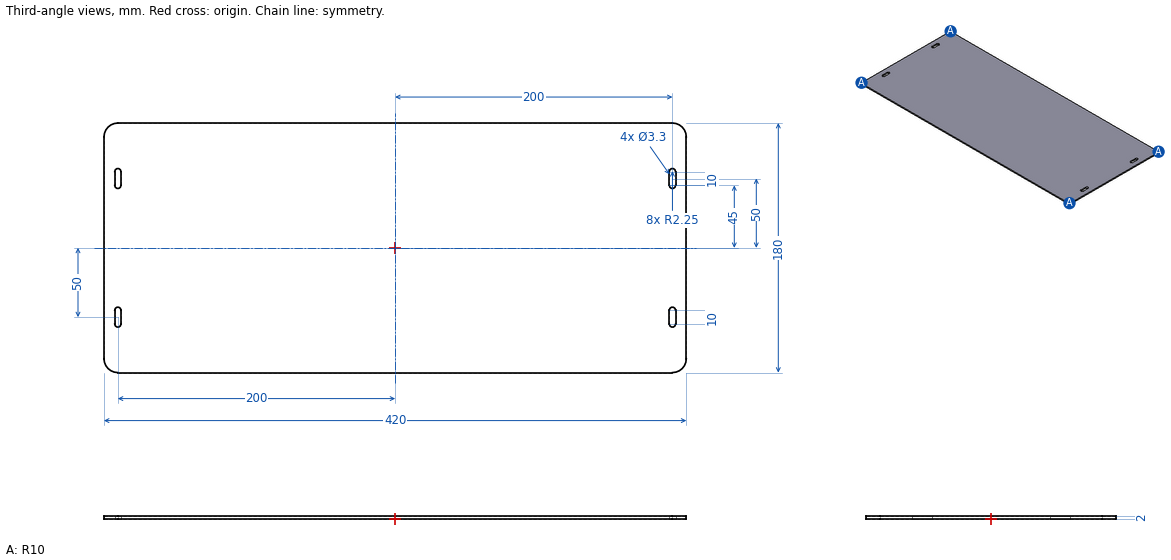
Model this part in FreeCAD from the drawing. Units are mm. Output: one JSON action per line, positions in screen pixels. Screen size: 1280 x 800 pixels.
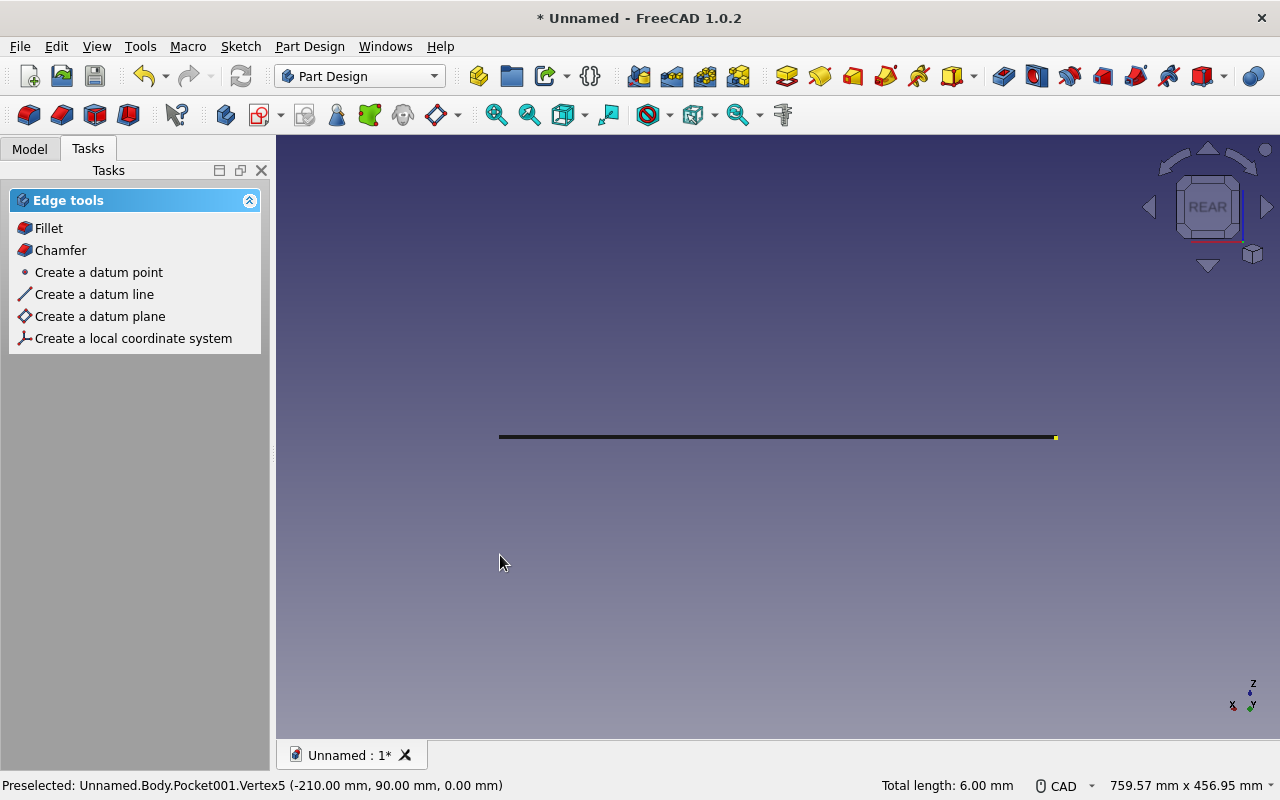
{"action": "scroll", "coordinate": [1056, 436], "scroll_direction": "up", "scroll_amount": 14}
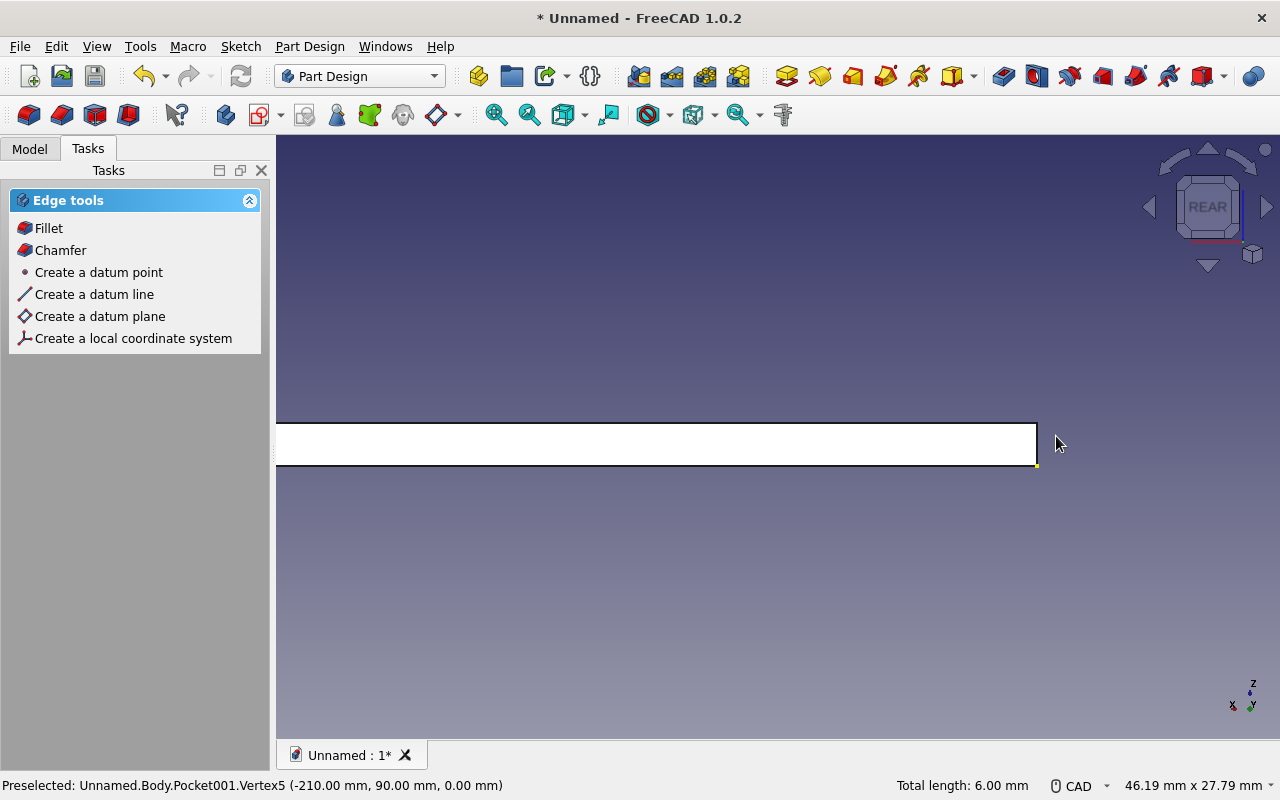
{"action": "left_click", "coordinate": [1037, 444], "text": "ctrl"}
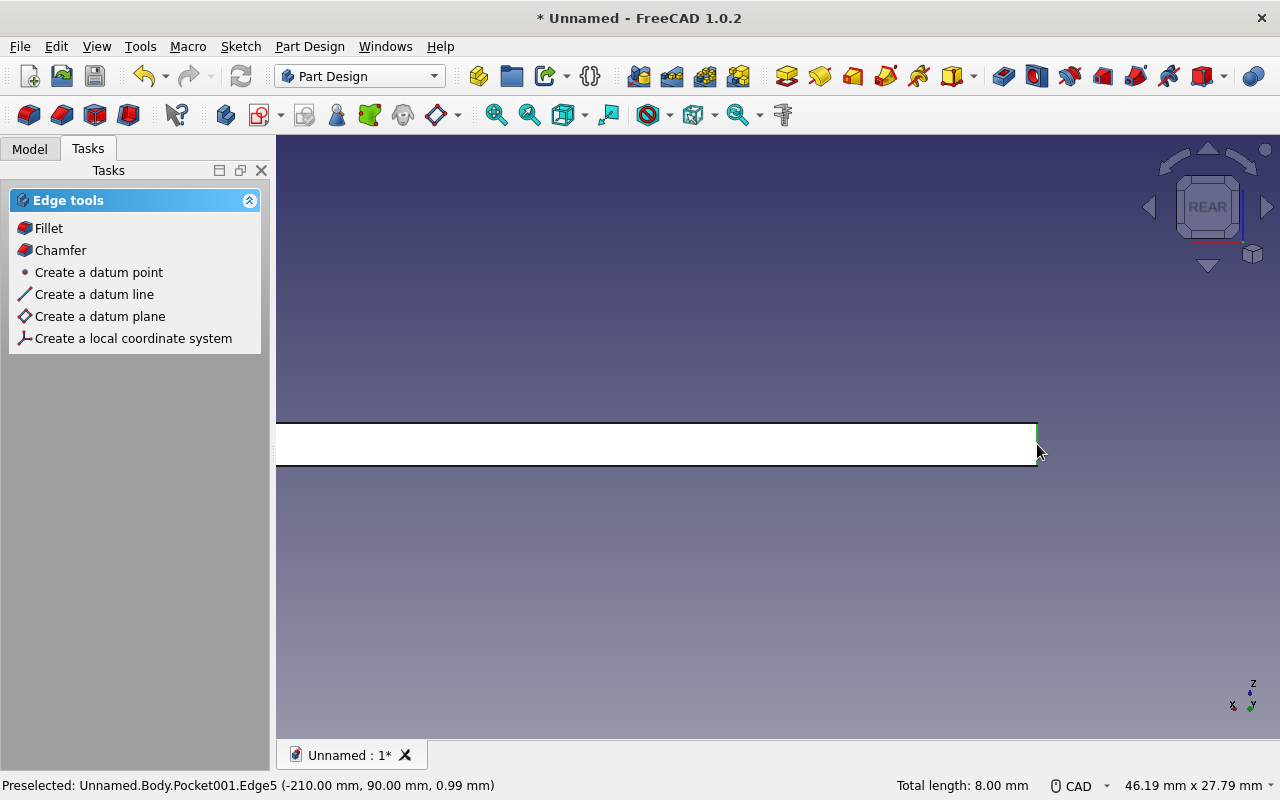
{"action": "left_click", "coordinate": [29, 116]}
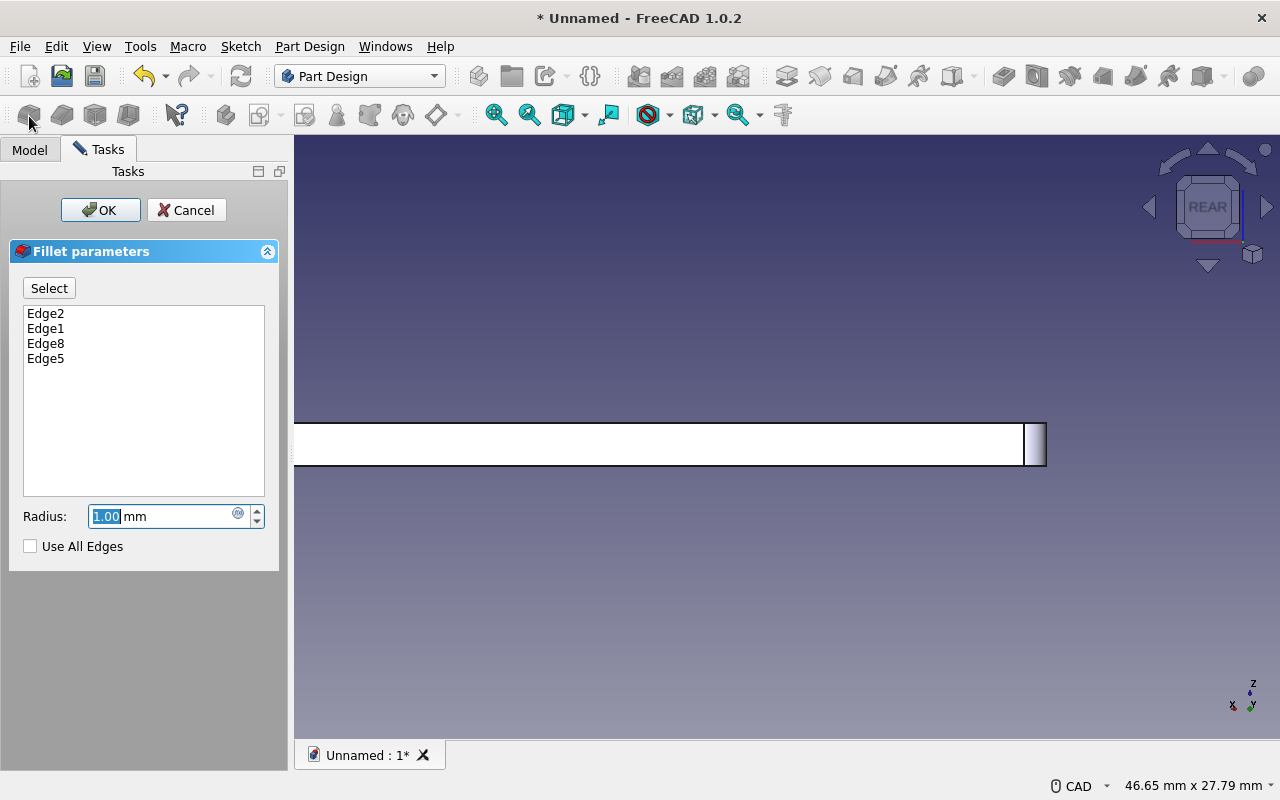
{"action": "type", "text": "10"}
{"action": "key", "text": "Tab"}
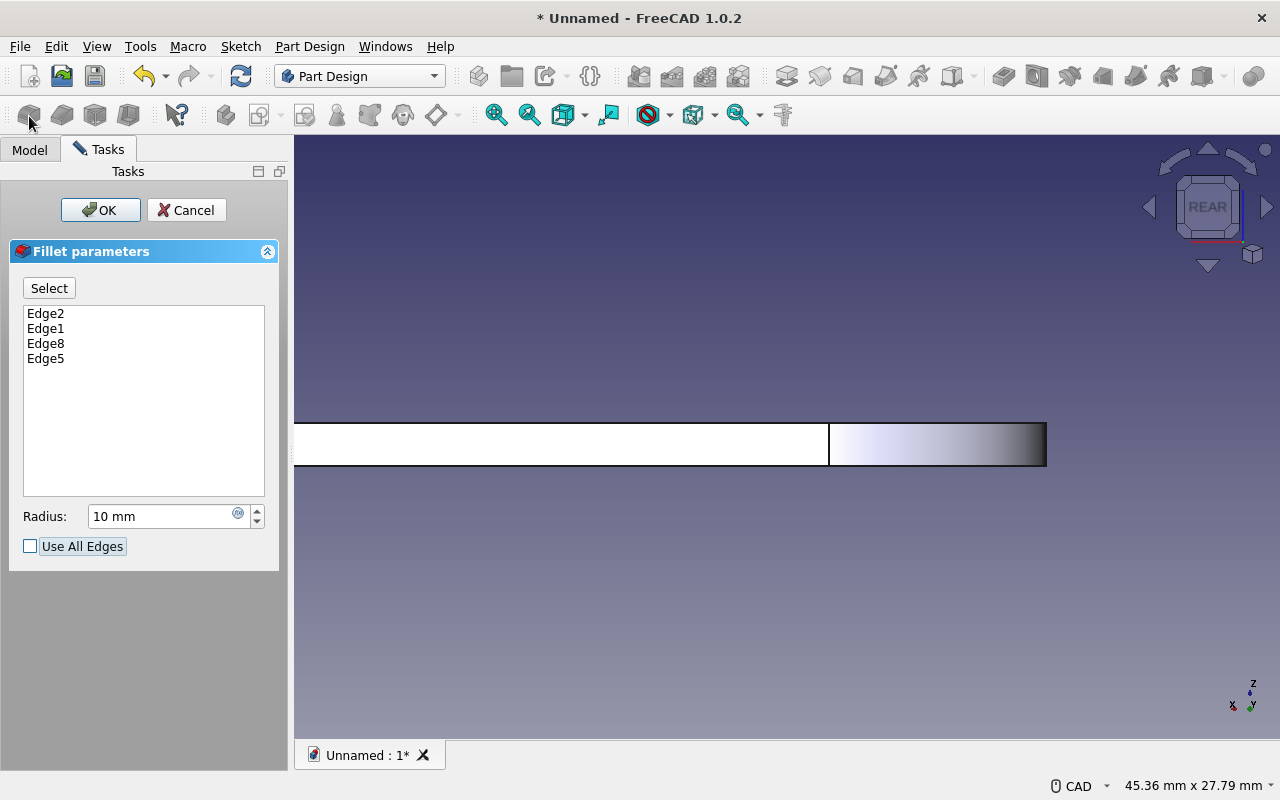
{"action": "left_click", "coordinate": [101, 210]}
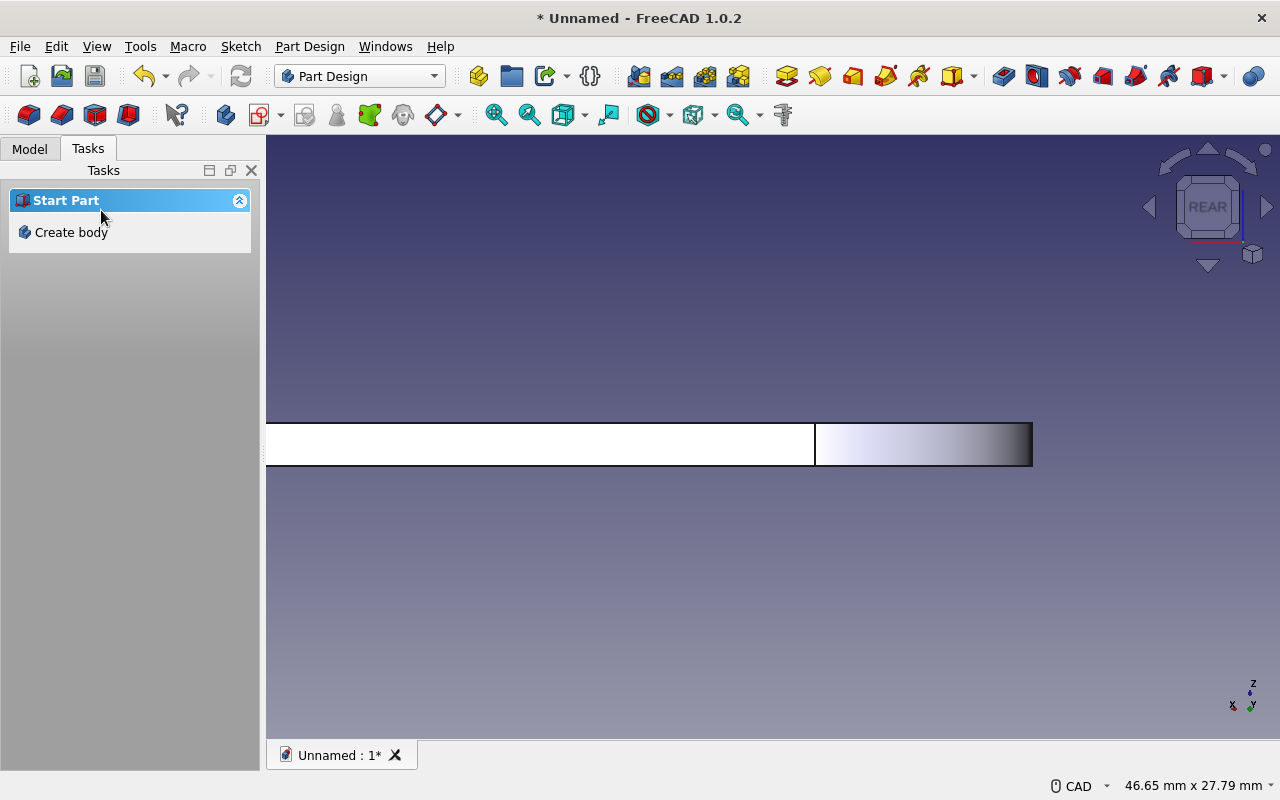
{"action": "key", "text": "0"}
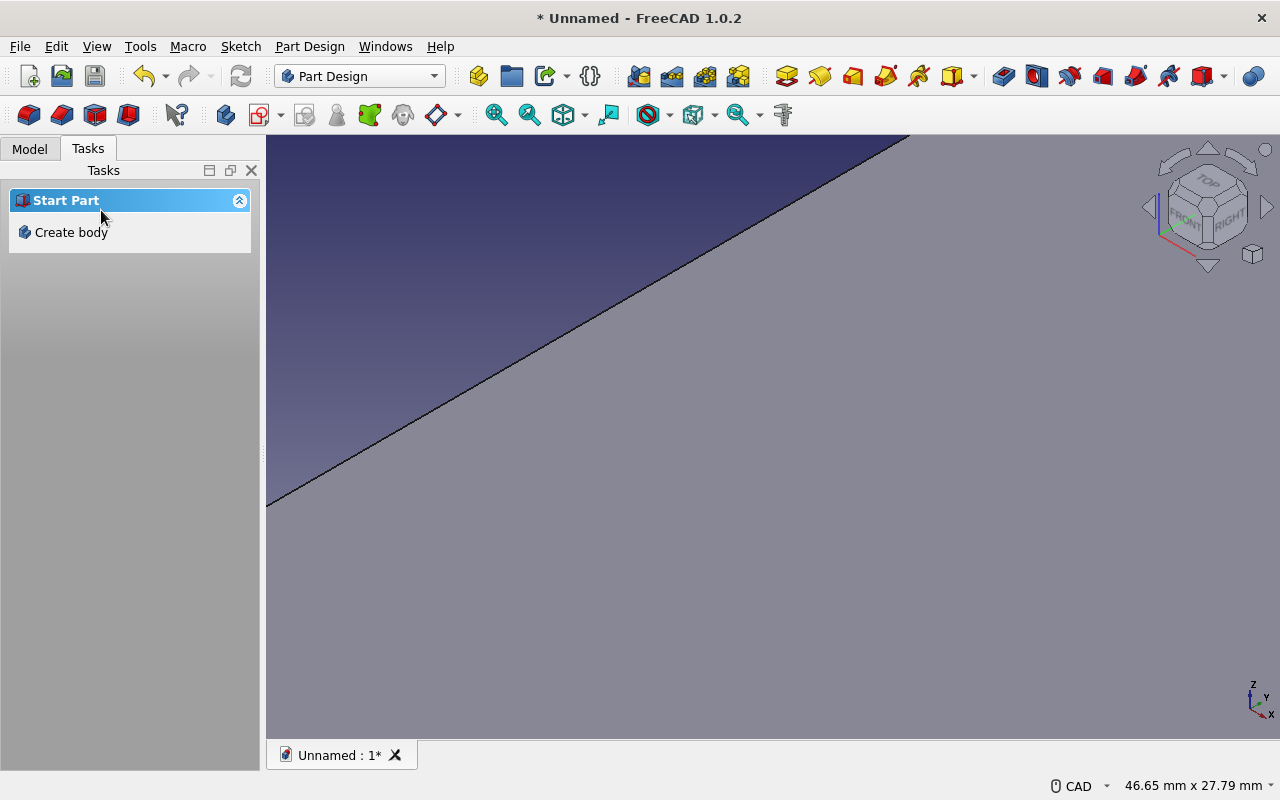
{"action": "key", "text": "v f"}